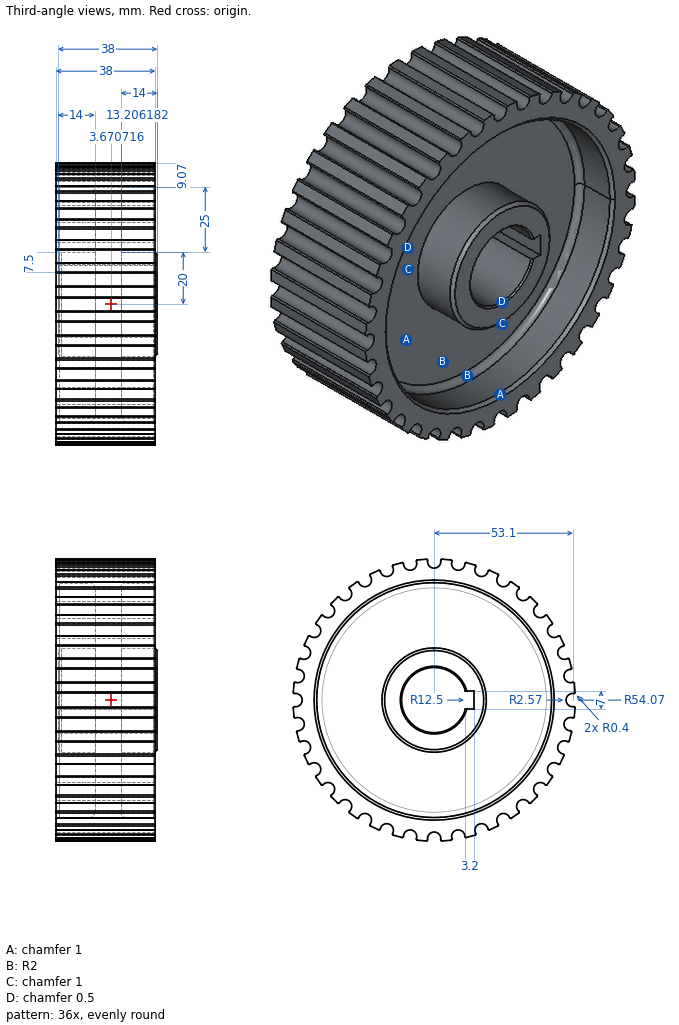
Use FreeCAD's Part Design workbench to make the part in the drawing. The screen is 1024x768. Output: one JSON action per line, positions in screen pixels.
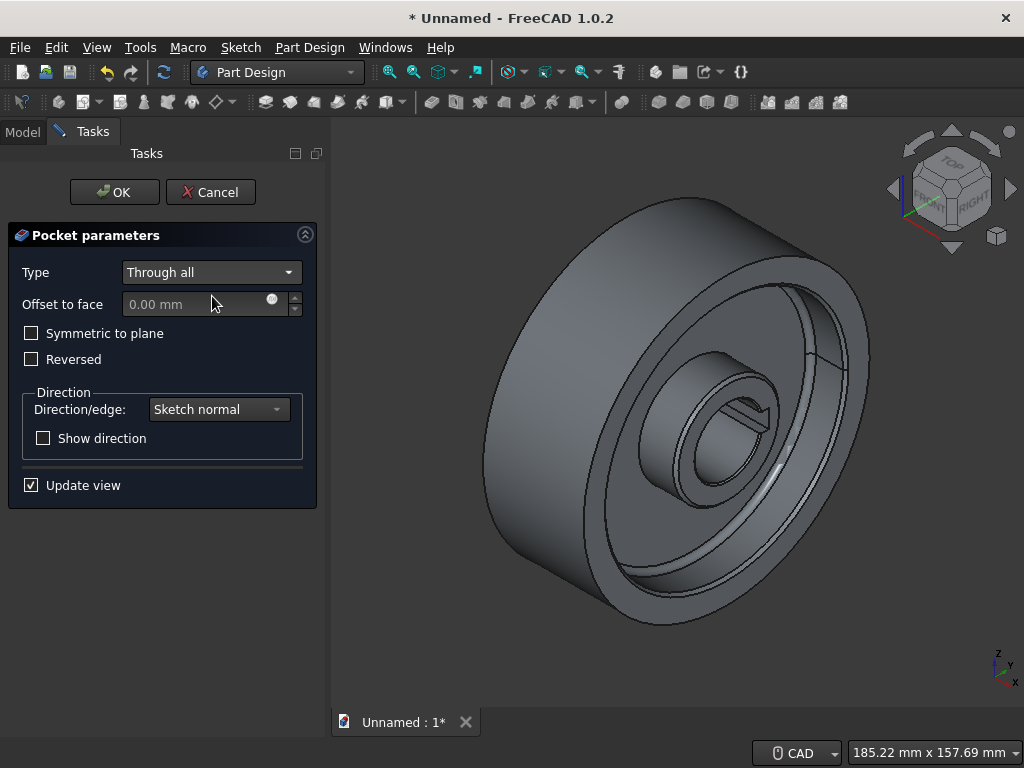
{"action": "left_click", "coordinate": [115, 192]}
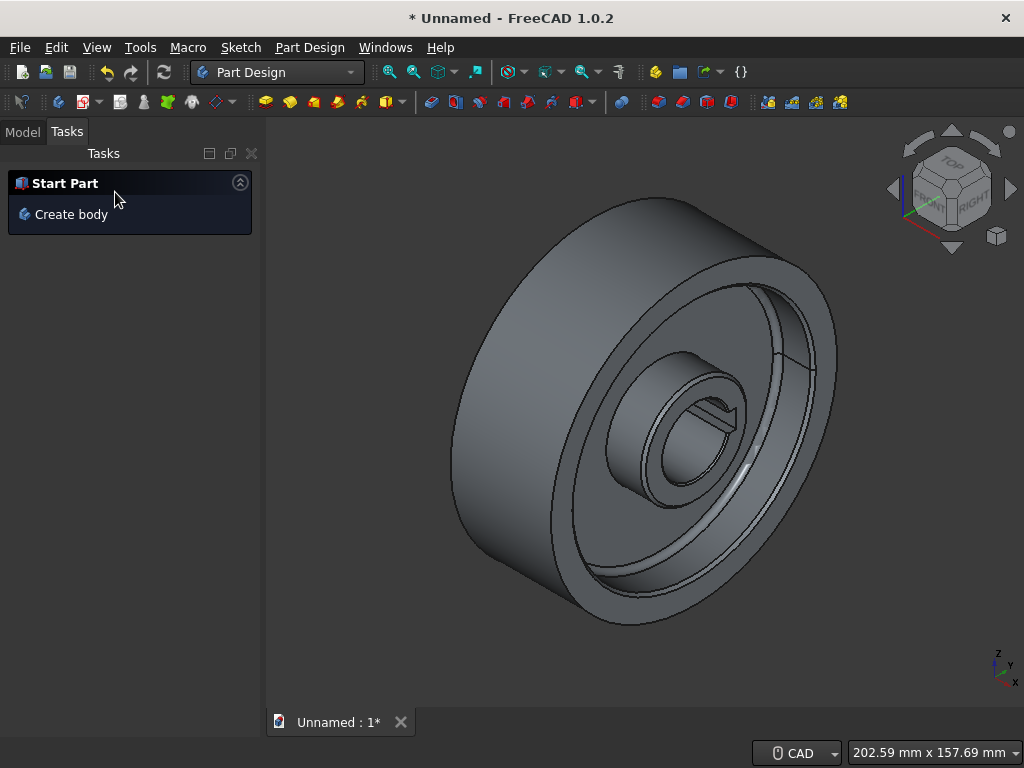
{"action": "key", "text": "6"}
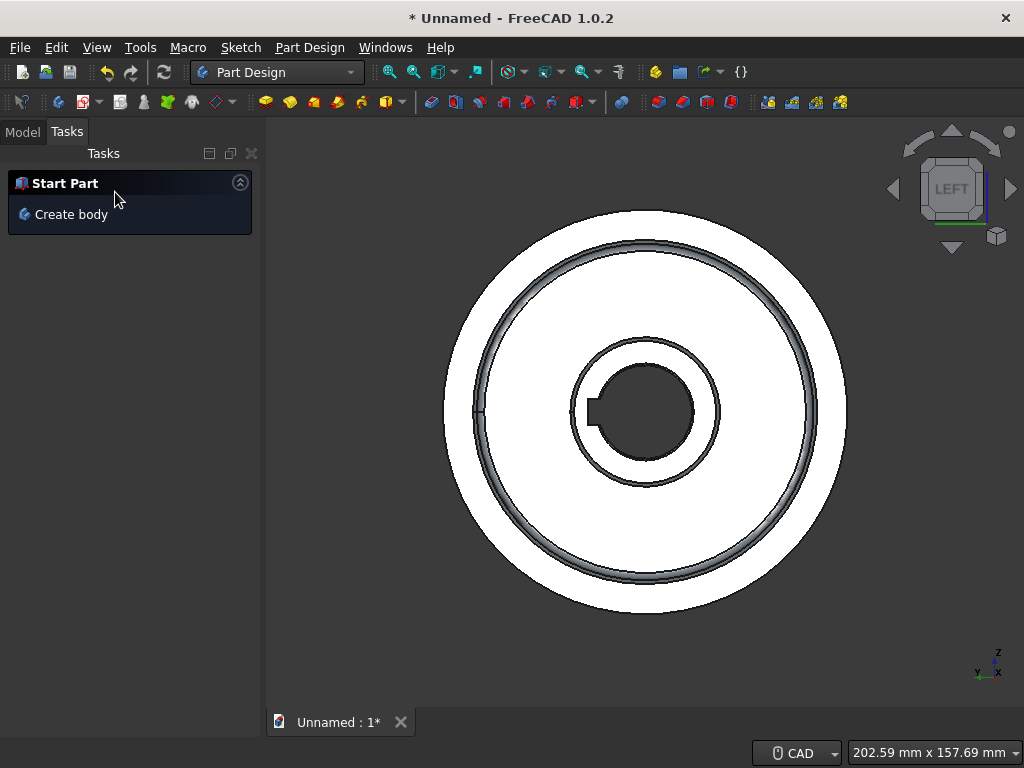
{"action": "left_click", "coordinate": [587, 238]}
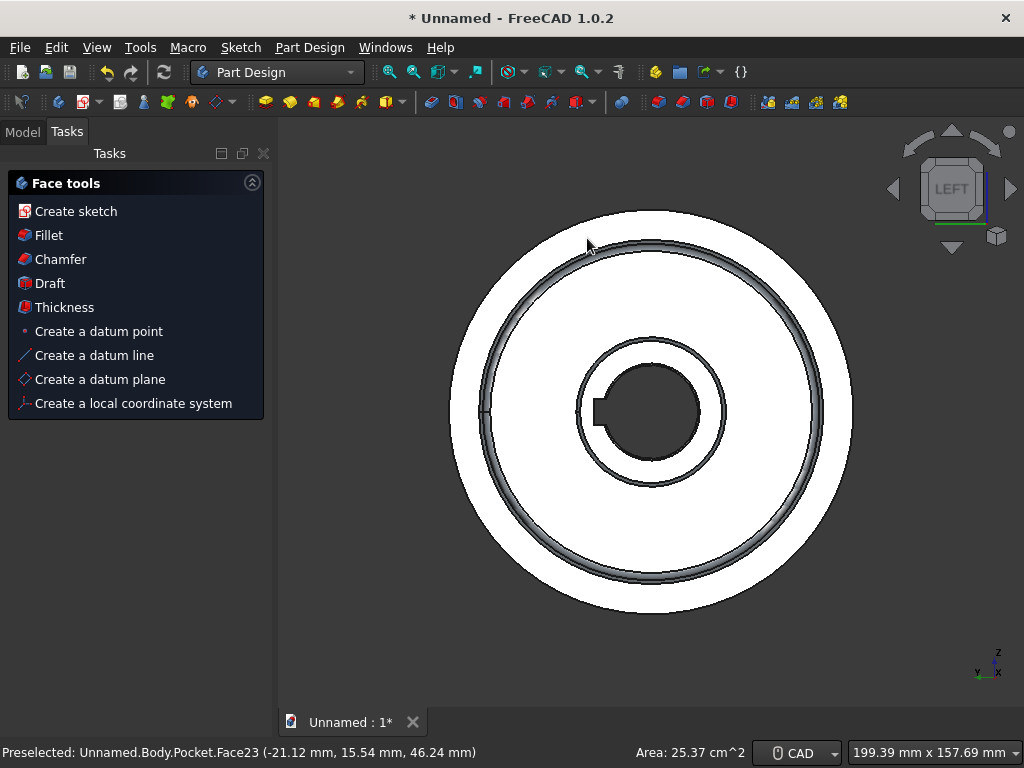
{"action": "left_click", "coordinate": [84, 102]}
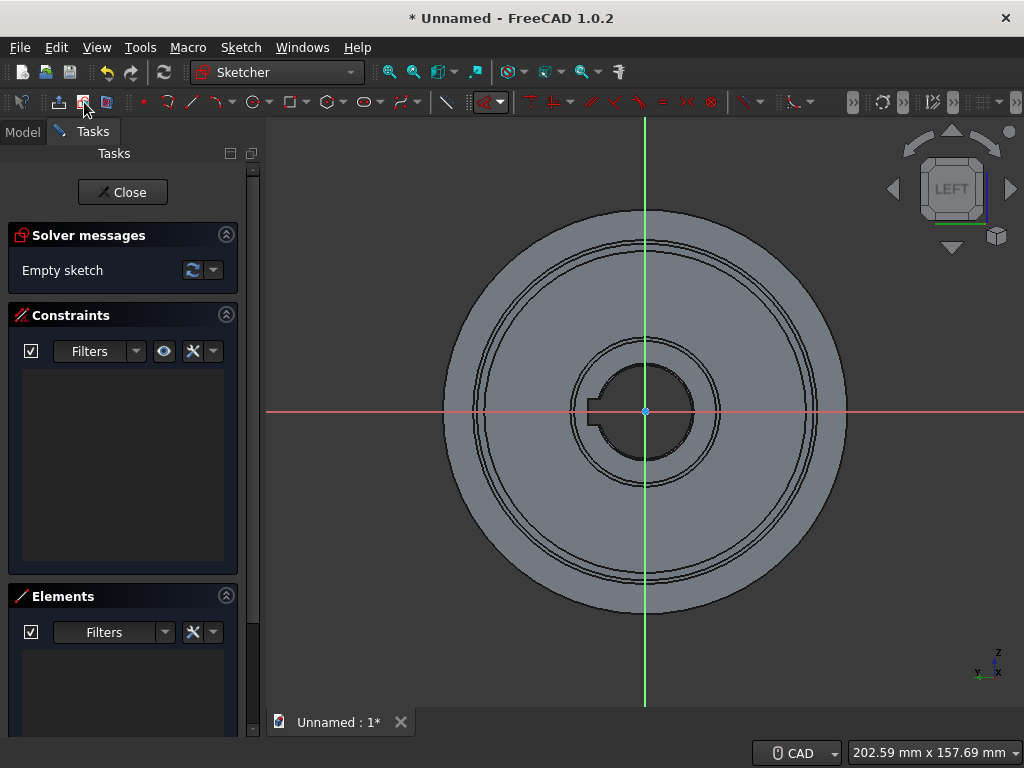
{"action": "scroll", "coordinate": [441, 412], "scroll_direction": "up", "scroll_amount": 14}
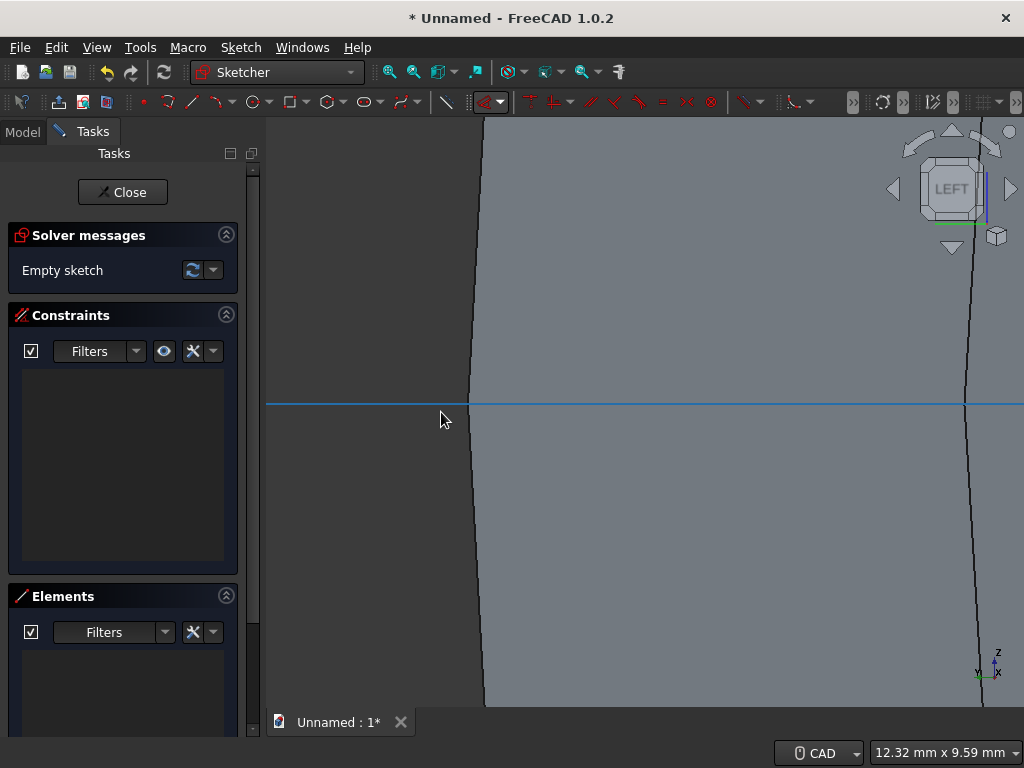
{"action": "left_click", "coordinate": [216, 102]}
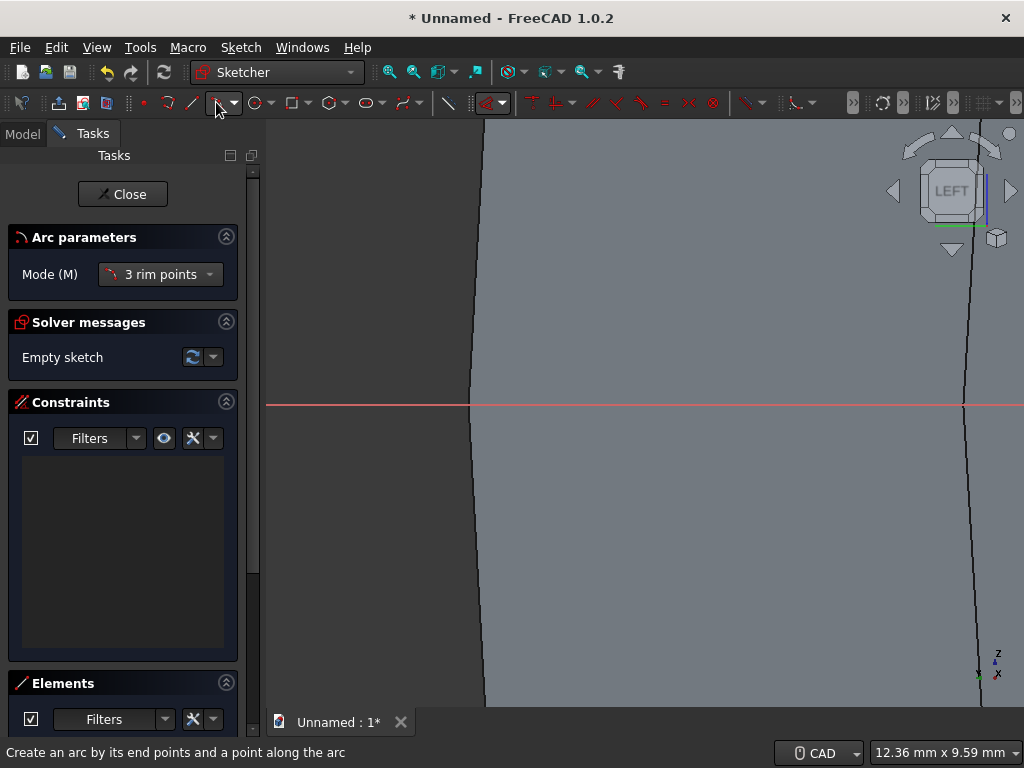
{"action": "left_click", "coordinate": [502, 561]}
{"action": "left_click", "coordinate": [502, 250]}
{"action": "left_click", "coordinate": [676, 459]}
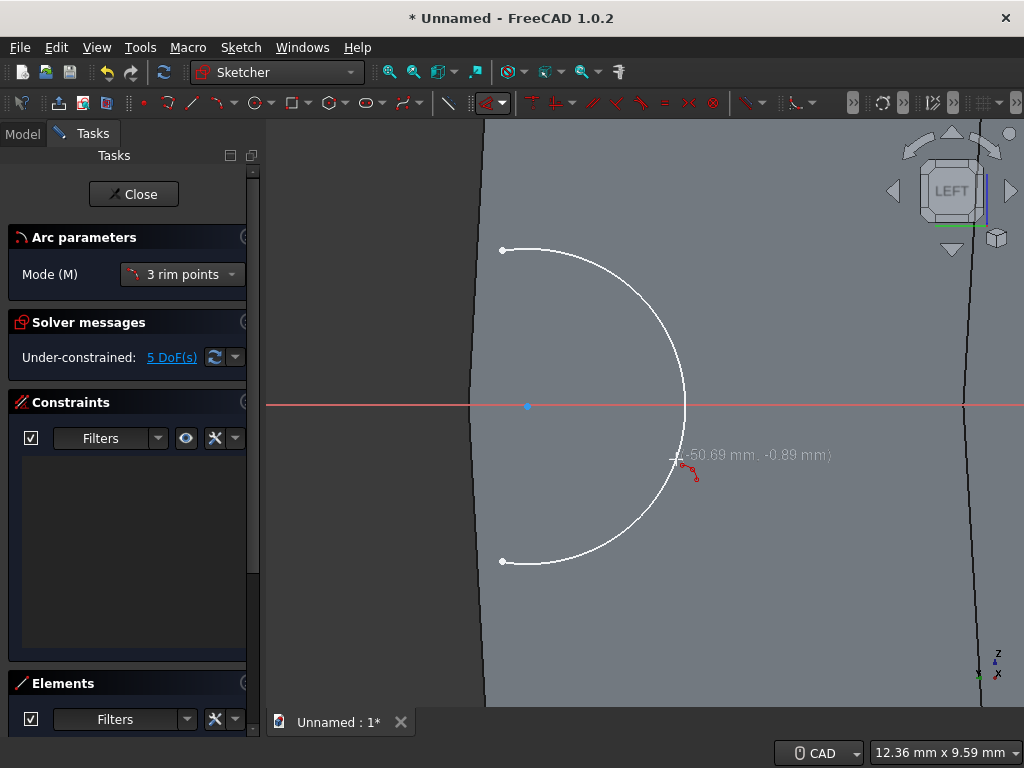
{"action": "left_click", "coordinate": [502, 251]}
{"action": "left_click", "coordinate": [473, 224]}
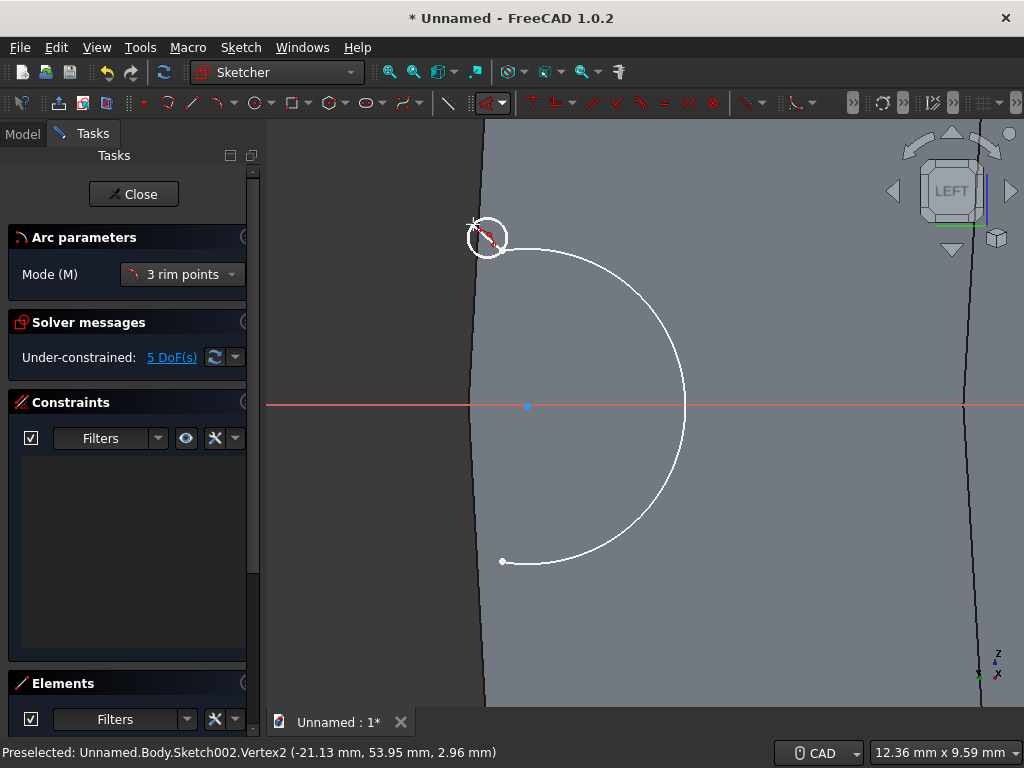
{"action": "scroll", "coordinate": [482, 244], "scroll_direction": "up", "scroll_amount": 3}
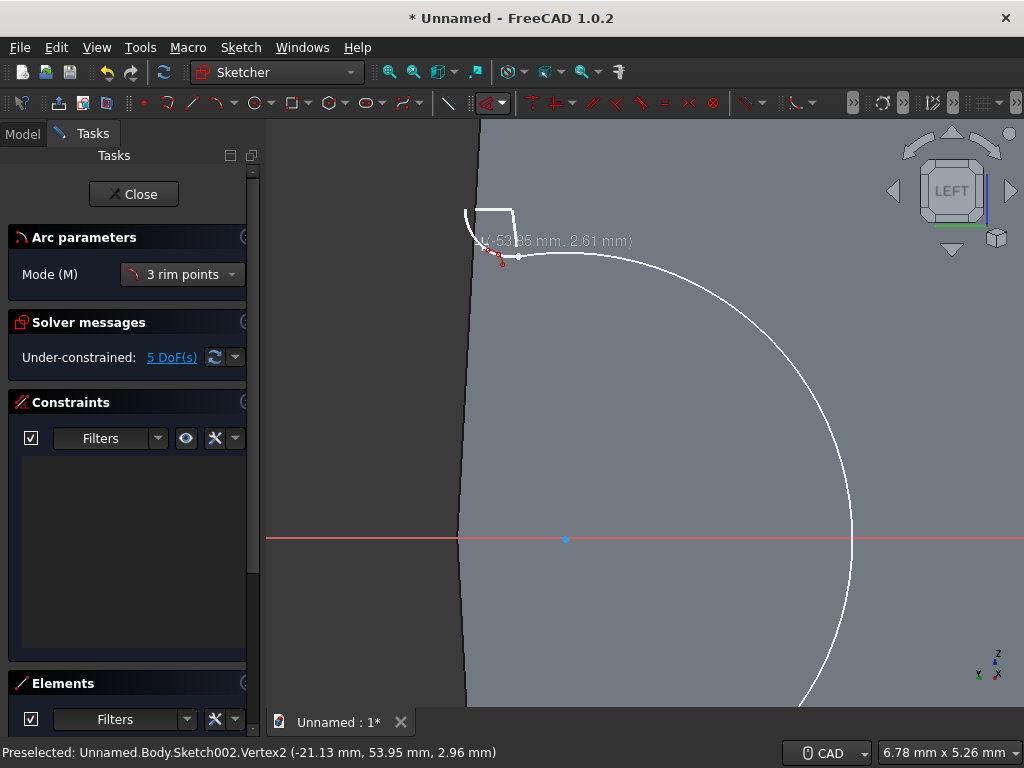
{"action": "left_click", "coordinate": [481, 244]}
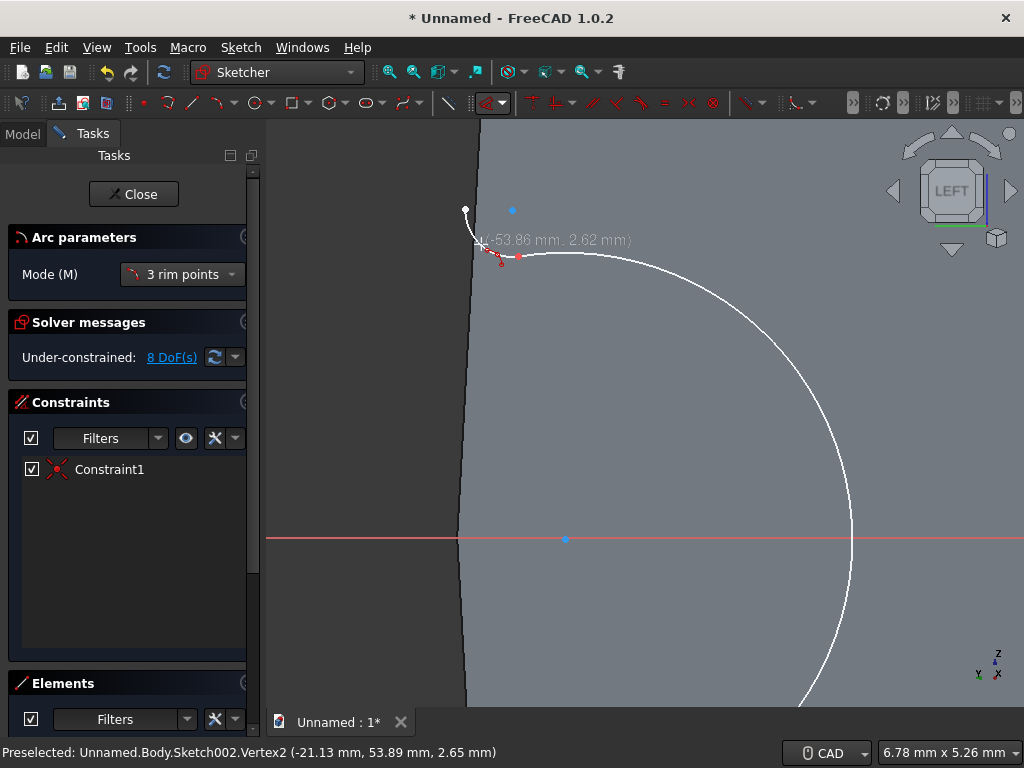
{"action": "left_click", "coordinate": [465, 209]}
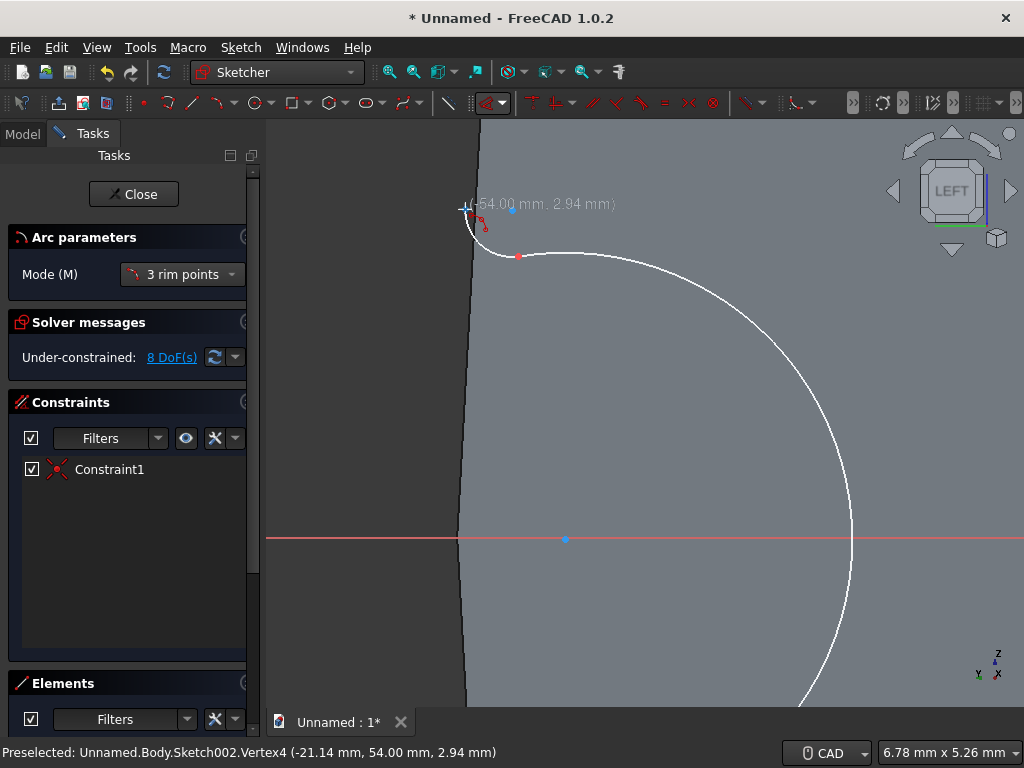
{"action": "scroll", "coordinate": [481, 261], "scroll_direction": "down", "scroll_amount": 3}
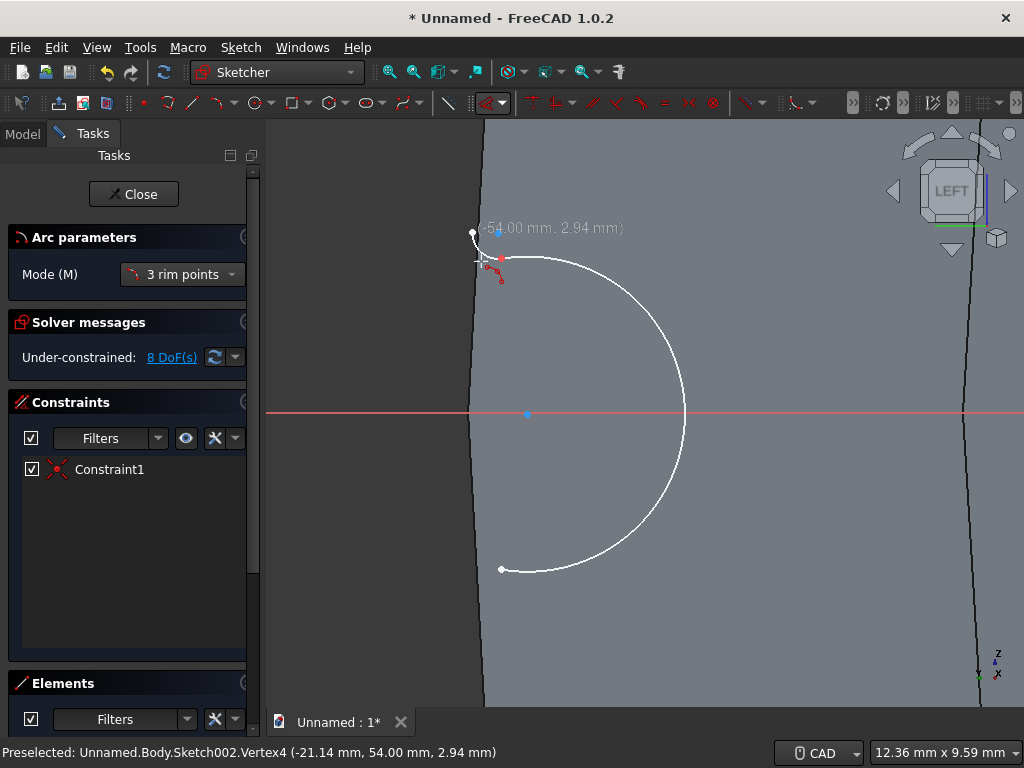
{"action": "left_click", "coordinate": [473, 594]}